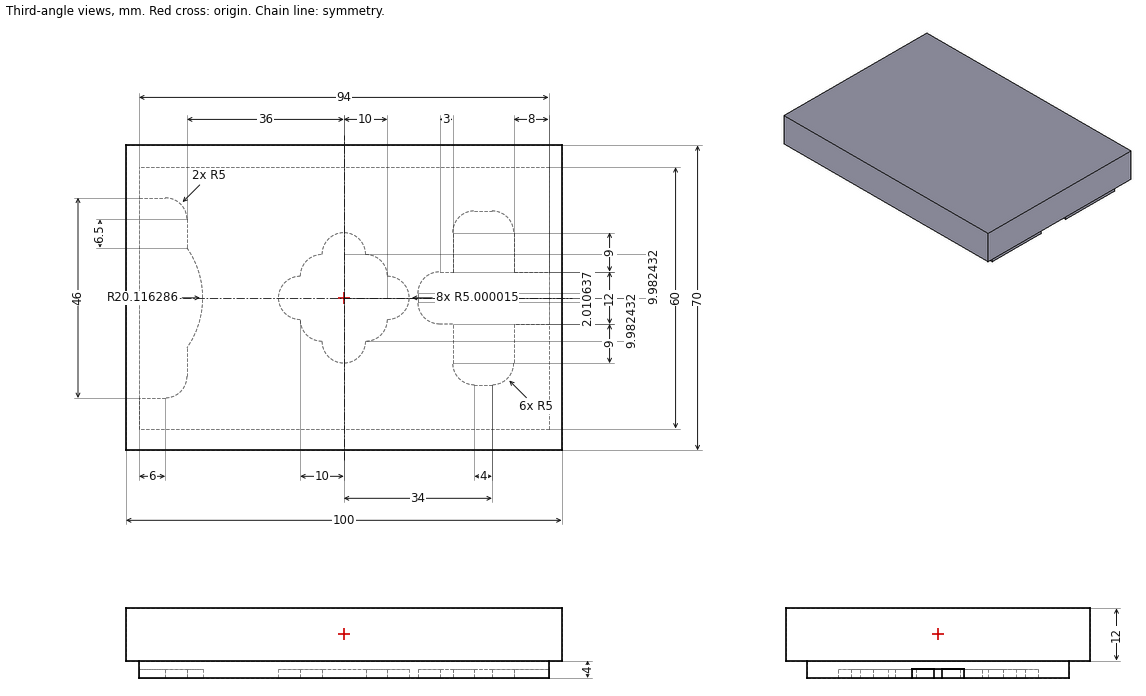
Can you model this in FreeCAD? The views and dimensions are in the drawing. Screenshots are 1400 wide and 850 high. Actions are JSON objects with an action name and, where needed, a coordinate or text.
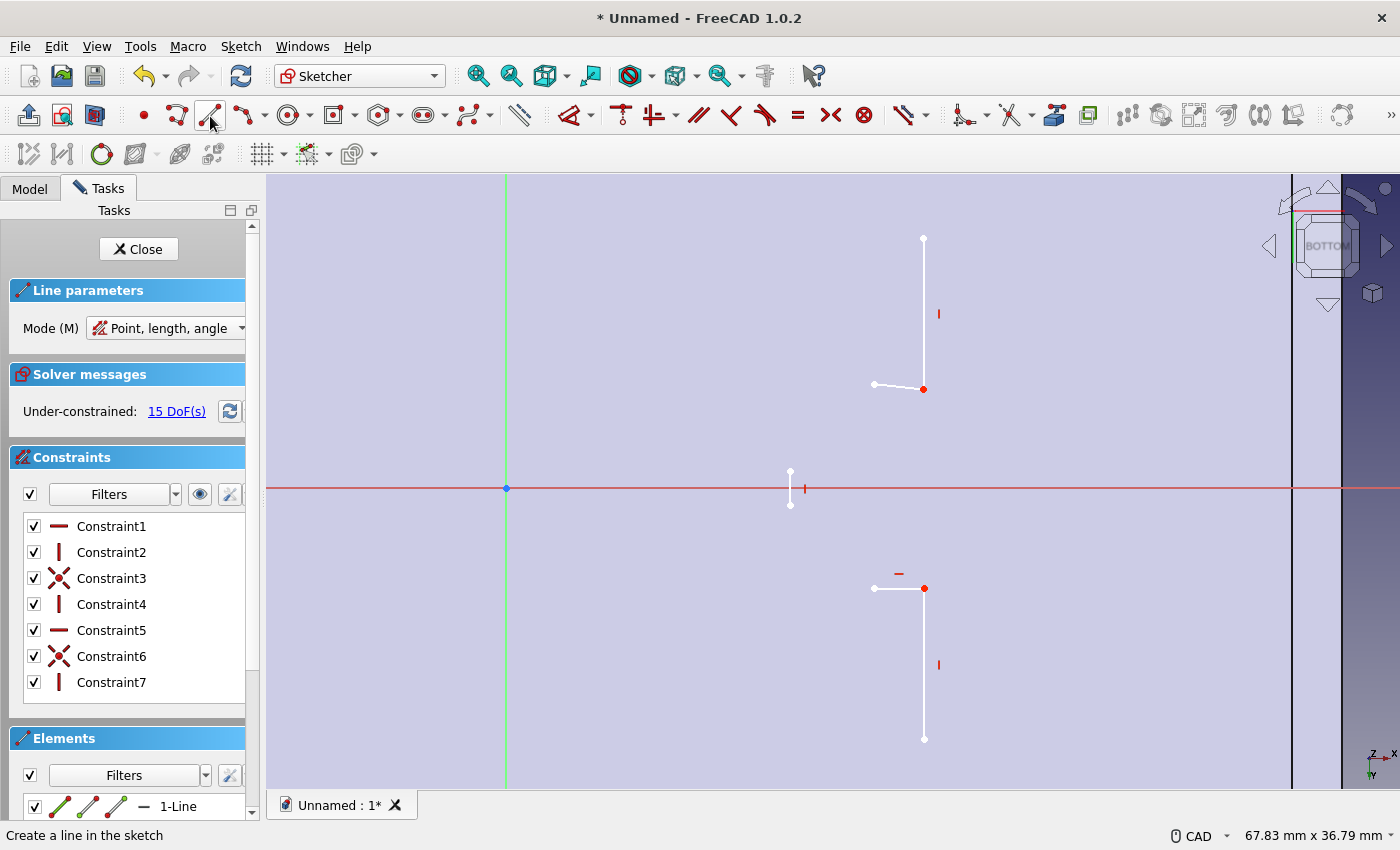
{"action": "scroll", "coordinate": [601, 474], "scroll_direction": "down", "scroll_amount": 3}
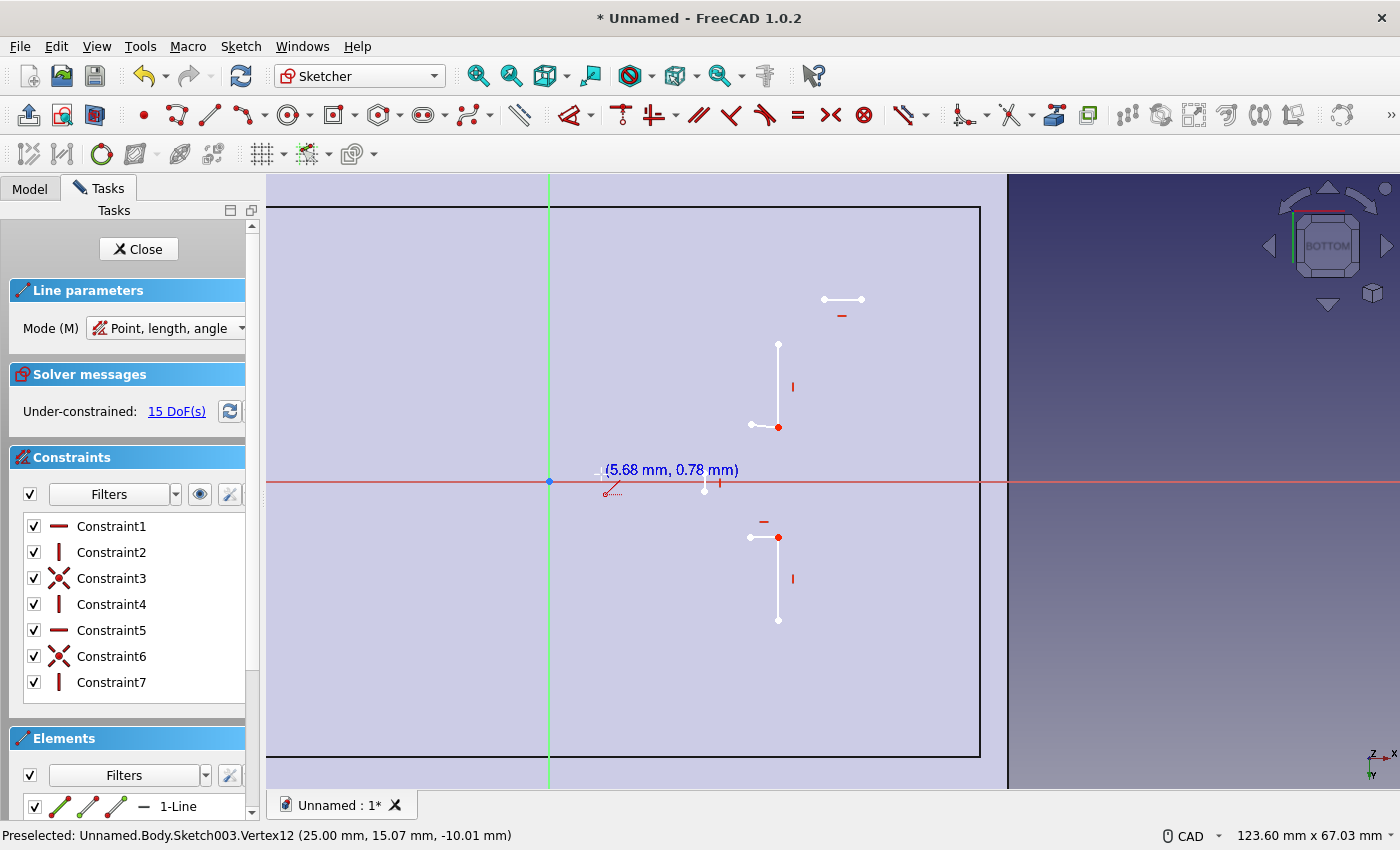
{"action": "left_click", "coordinate": [824, 665]}
{"action": "left_click", "coordinate": [861, 665]}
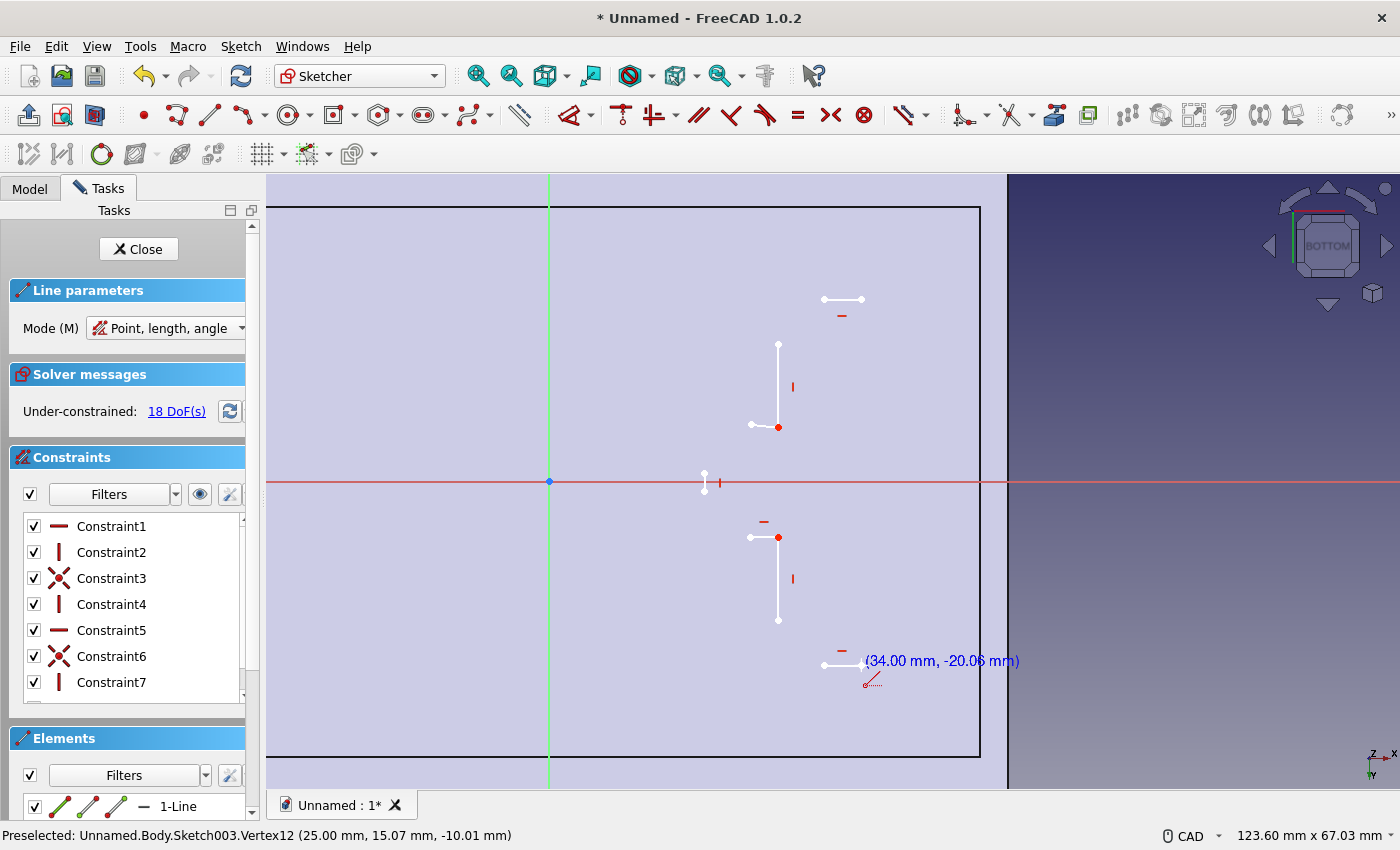
{"action": "left_click", "coordinate": [177, 116]}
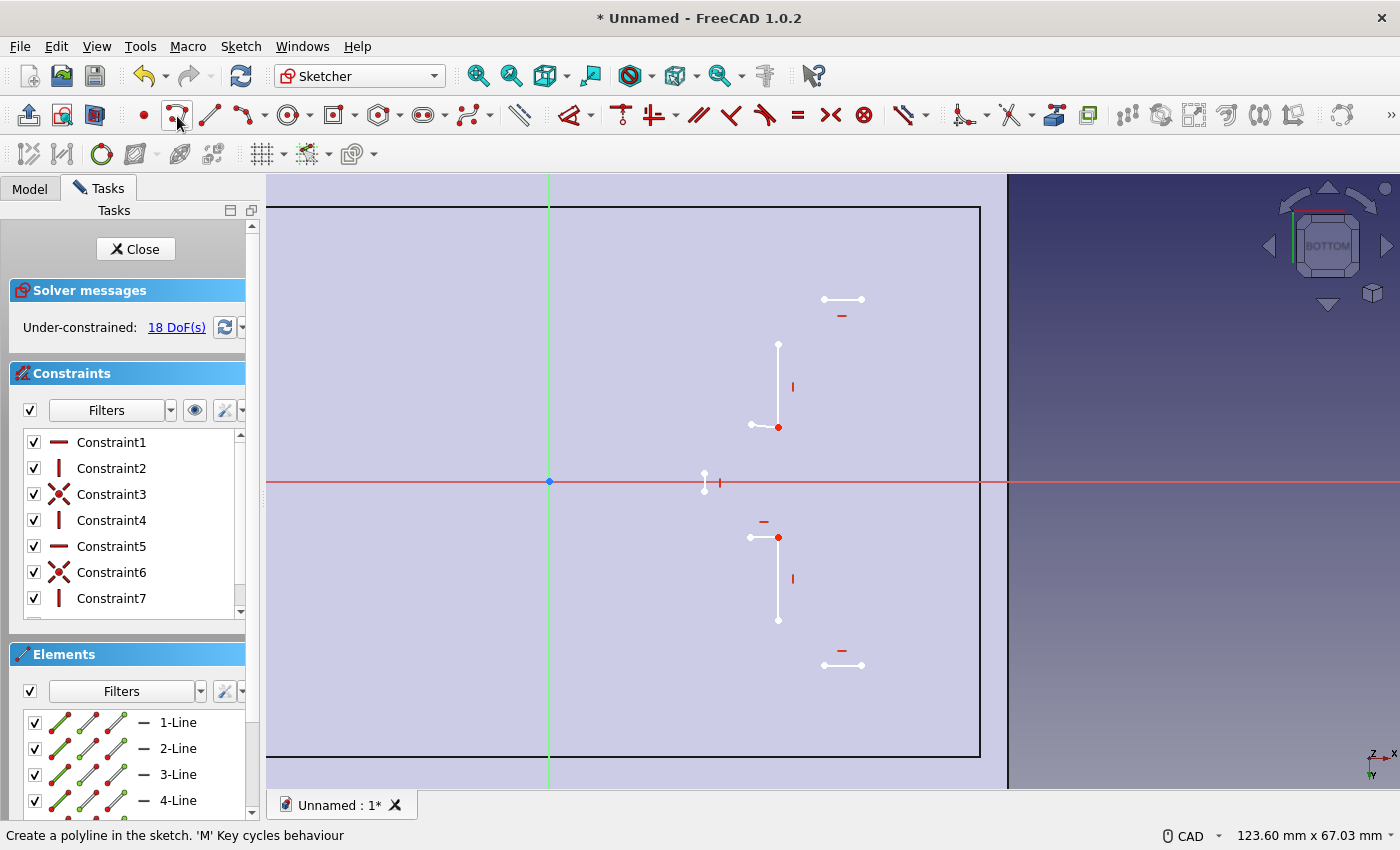
{"action": "left_click", "coordinate": [907, 620]}
{"action": "left_click", "coordinate": [907, 537]}
{"action": "left_click", "coordinate": [980, 537]}
{"action": "left_click", "coordinate": [980, 427]}
{"action": "left_click", "coordinate": [907, 427]}
{"action": "left_click", "coordinate": [907, 344]}
{"action": "right_click", "coordinate": [907, 344]}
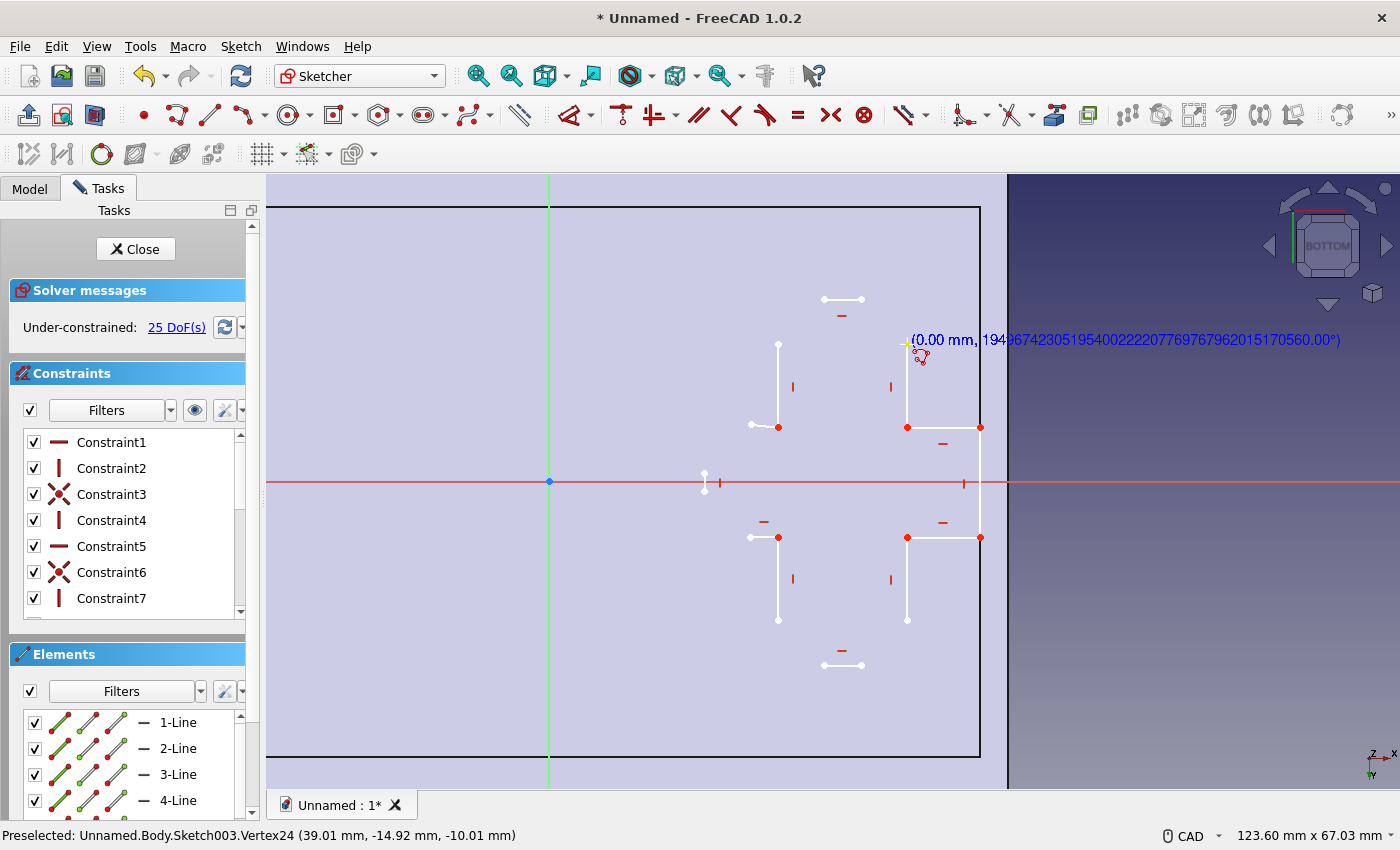
{"action": "left_click", "coordinate": [242, 116]}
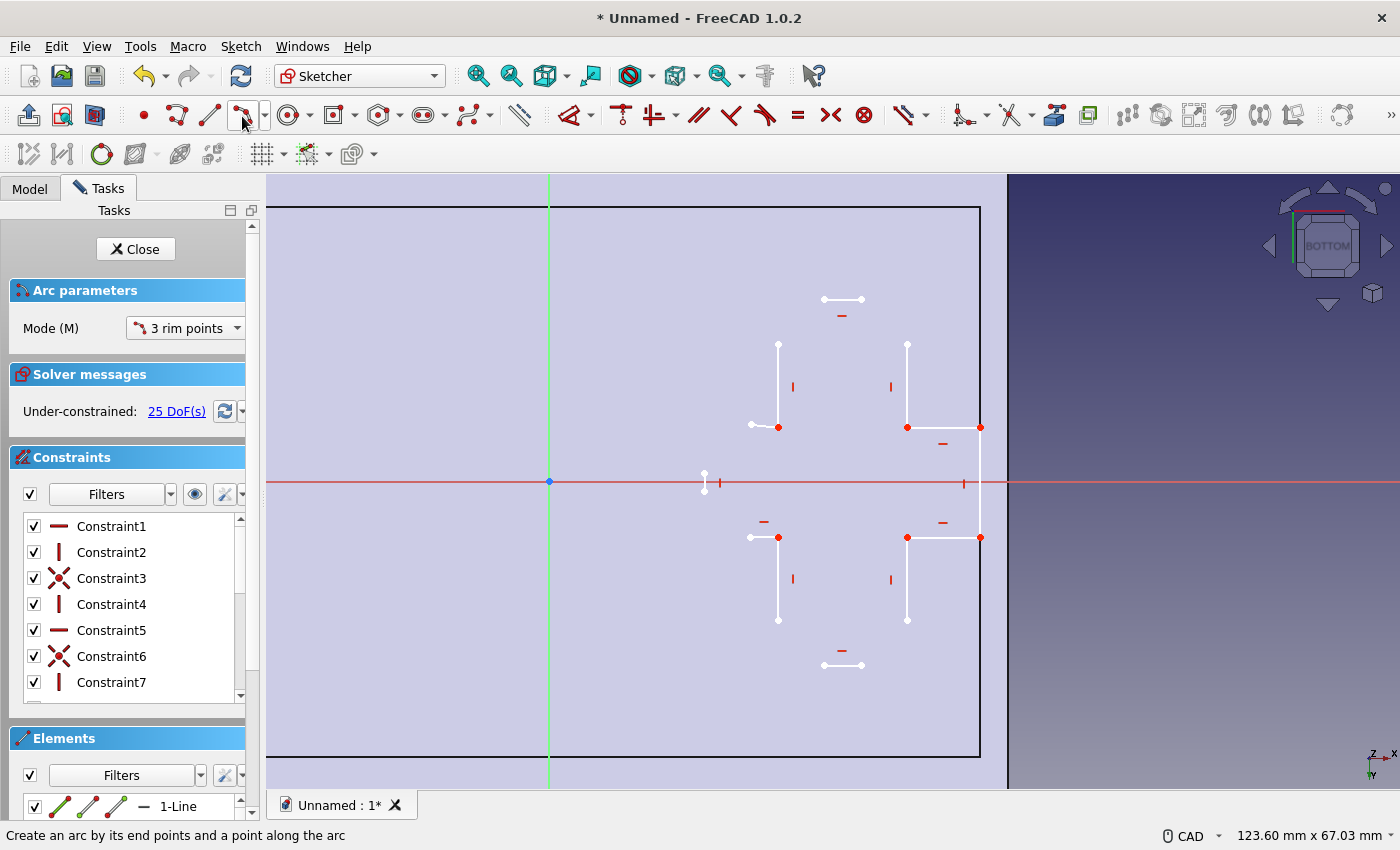
{"action": "left_click", "coordinate": [824, 300]}
{"action": "left_click", "coordinate": [778, 345]}
{"action": "left_click", "coordinate": [792, 312]}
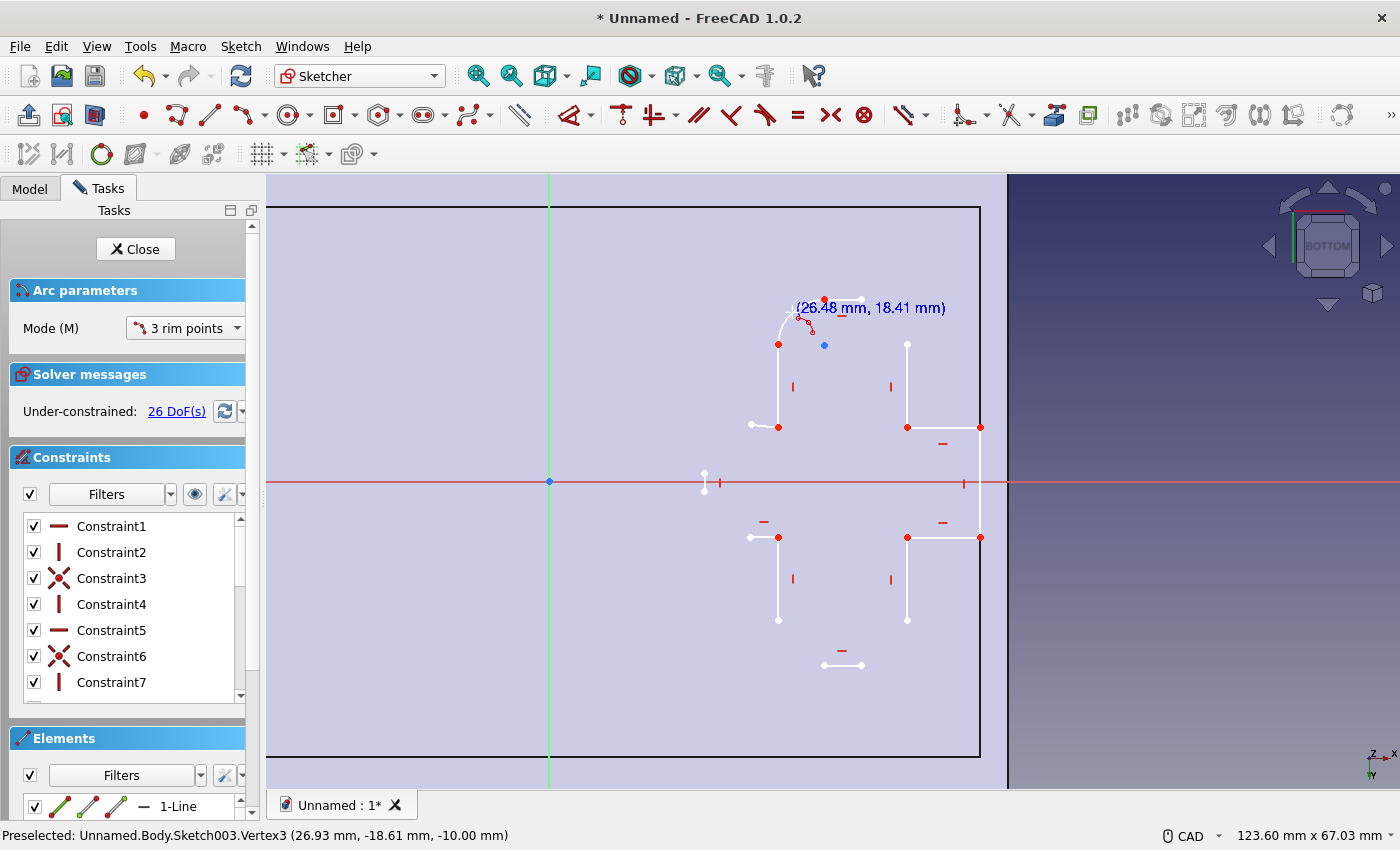
{"action": "left_click", "coordinate": [751, 425]}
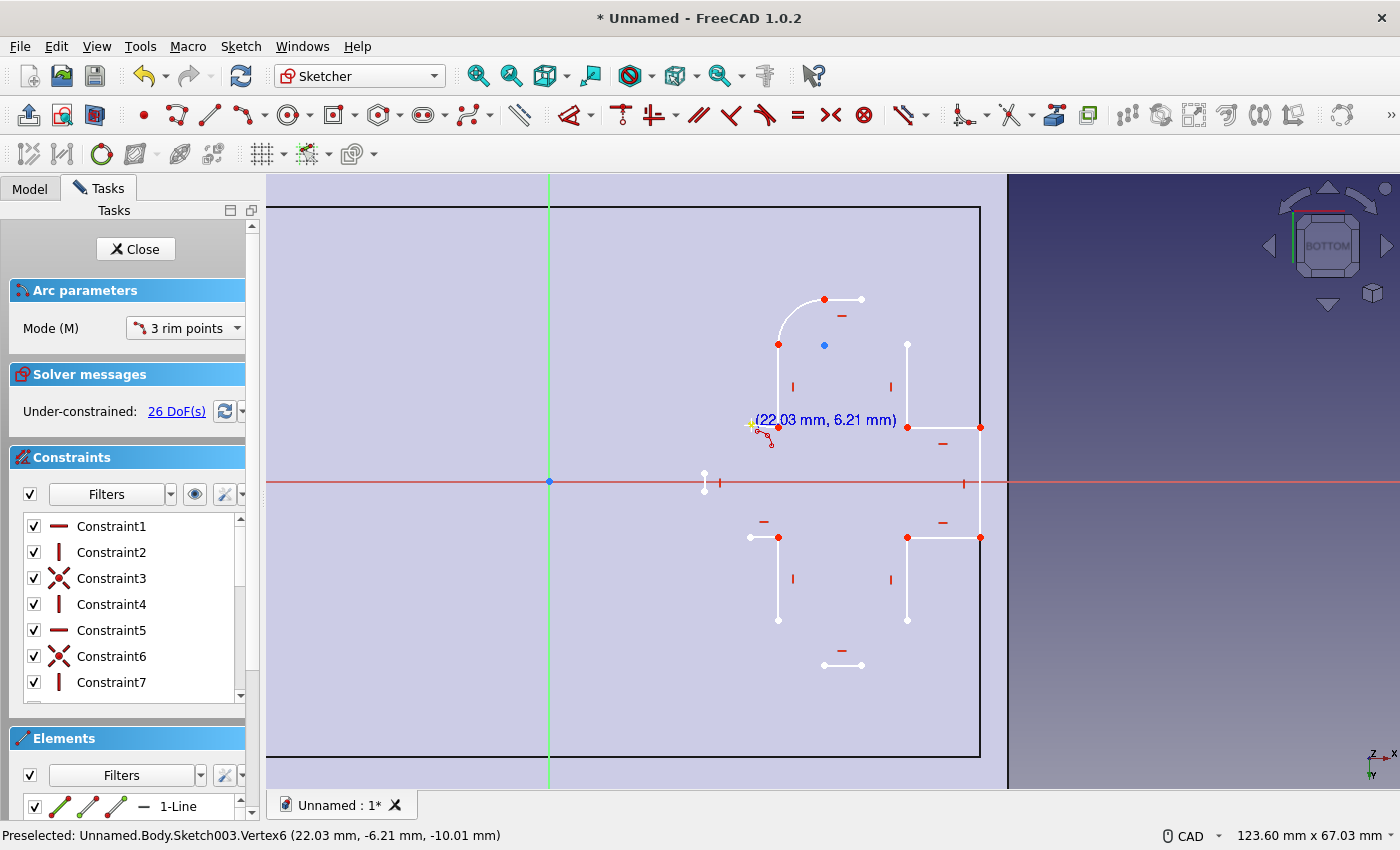
{"action": "scroll", "coordinate": [705, 473], "scroll_direction": "up", "scroll_amount": 3}